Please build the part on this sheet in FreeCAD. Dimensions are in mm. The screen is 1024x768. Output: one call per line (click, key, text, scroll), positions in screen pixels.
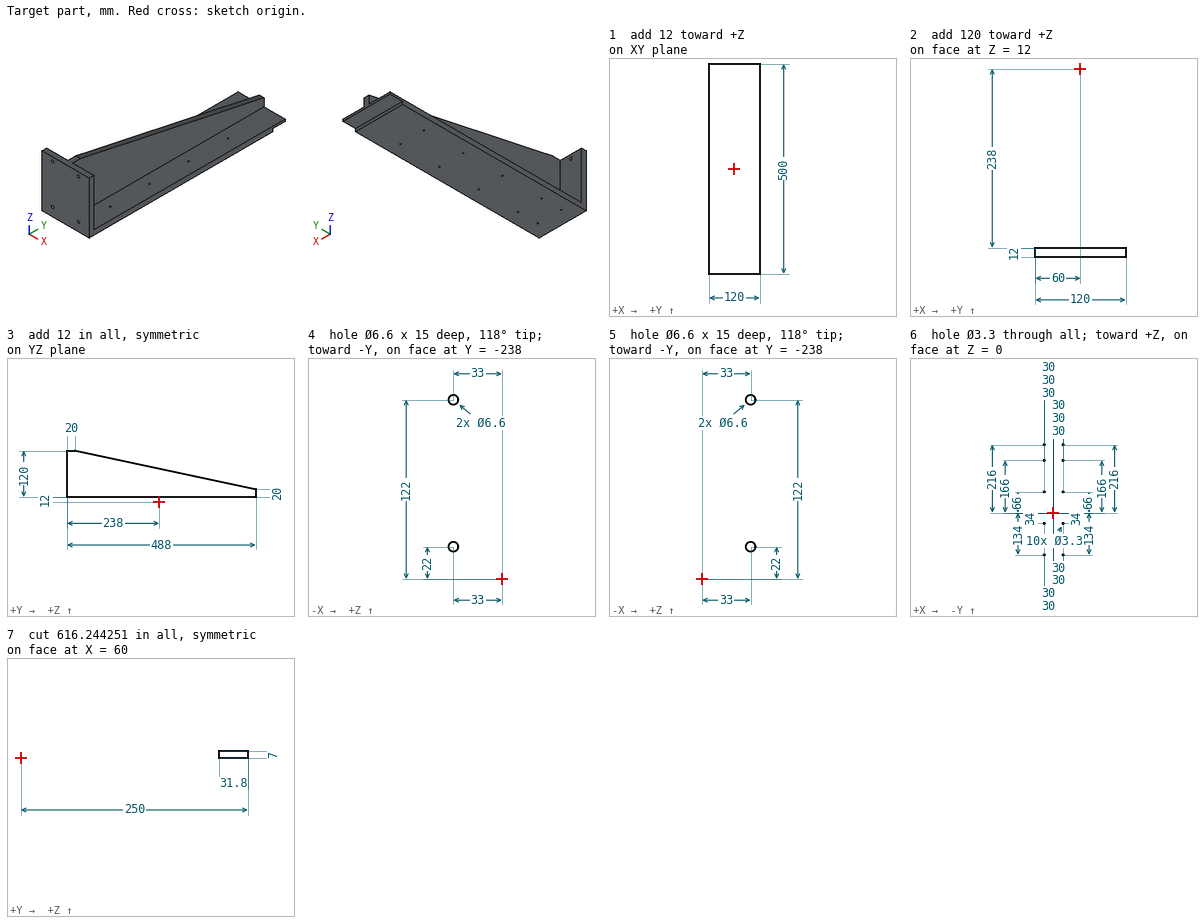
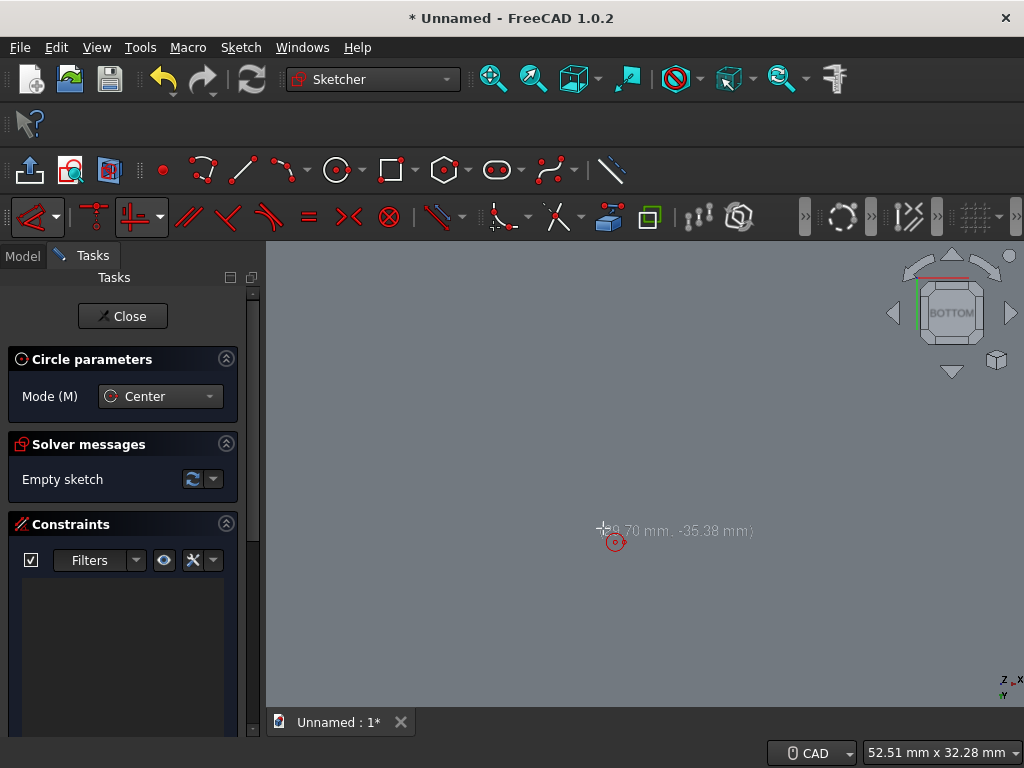
scroll(603, 541, down, 14)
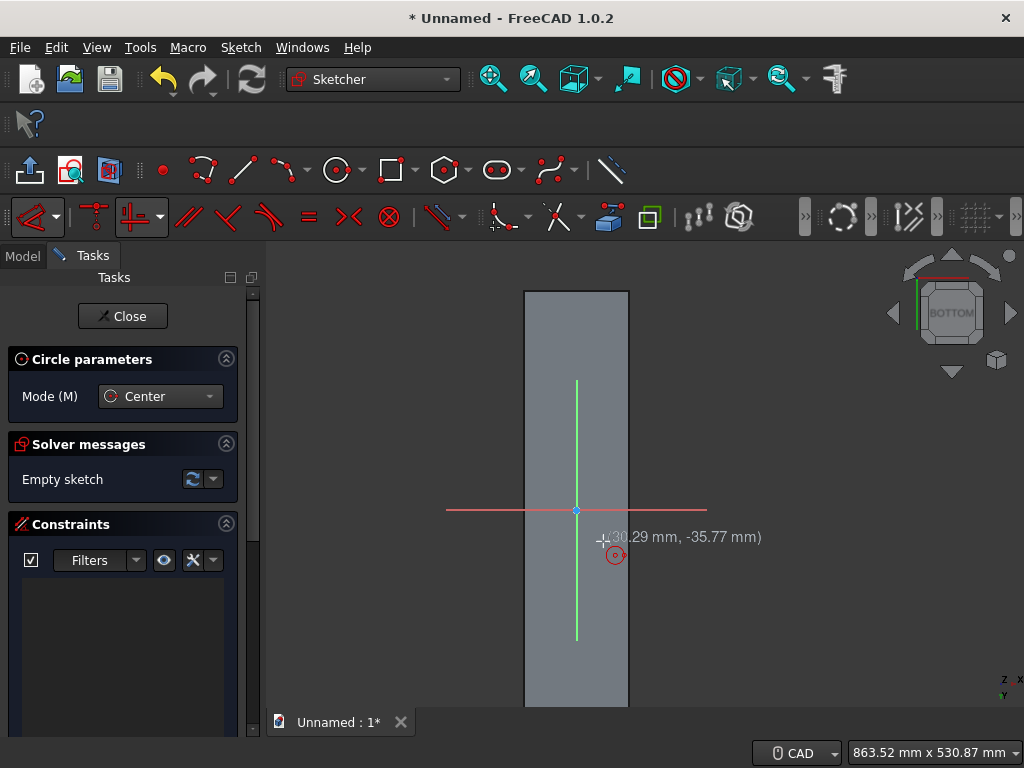
click(603, 540)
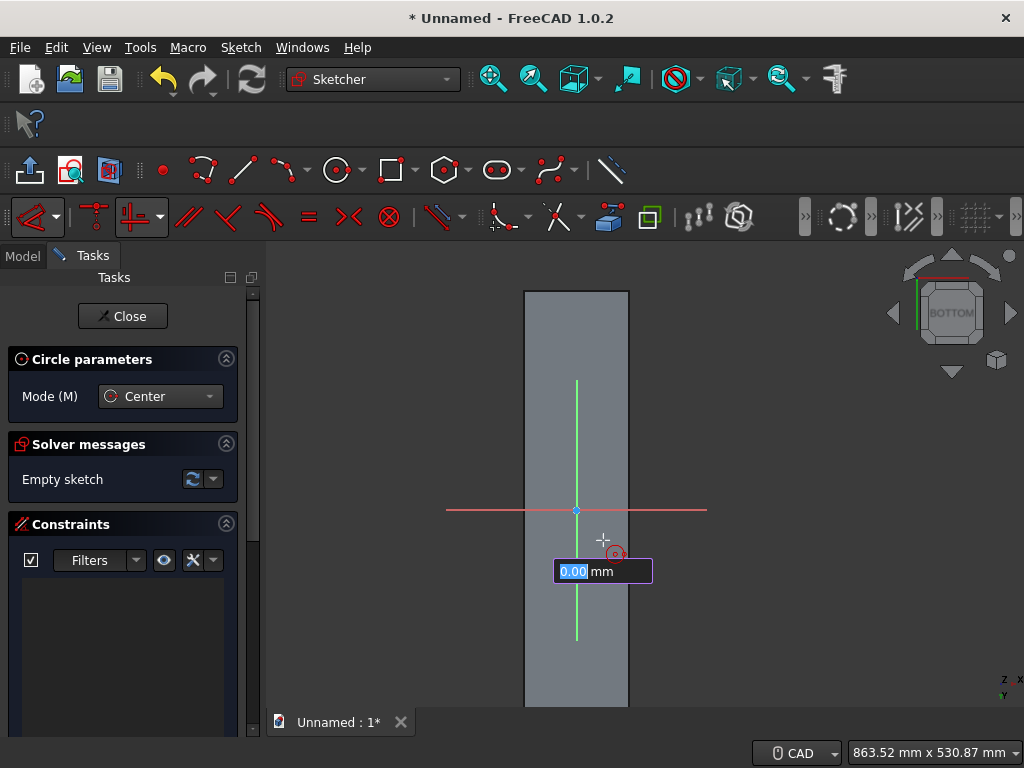
scroll(604, 539, up, 12)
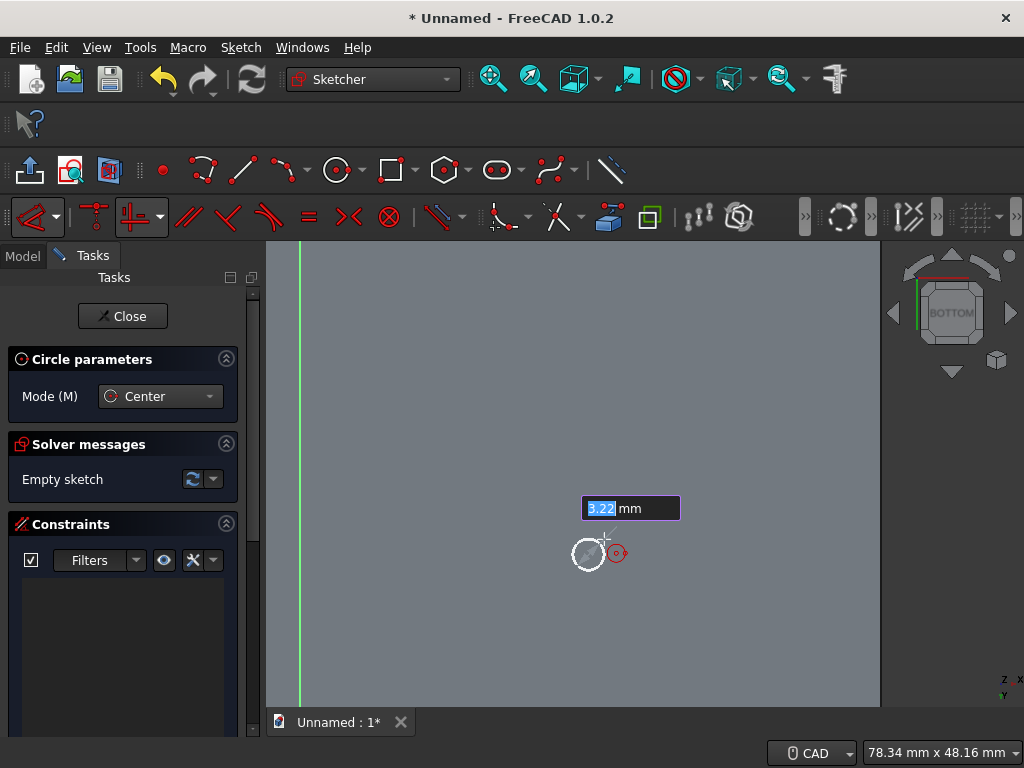
click(602, 534)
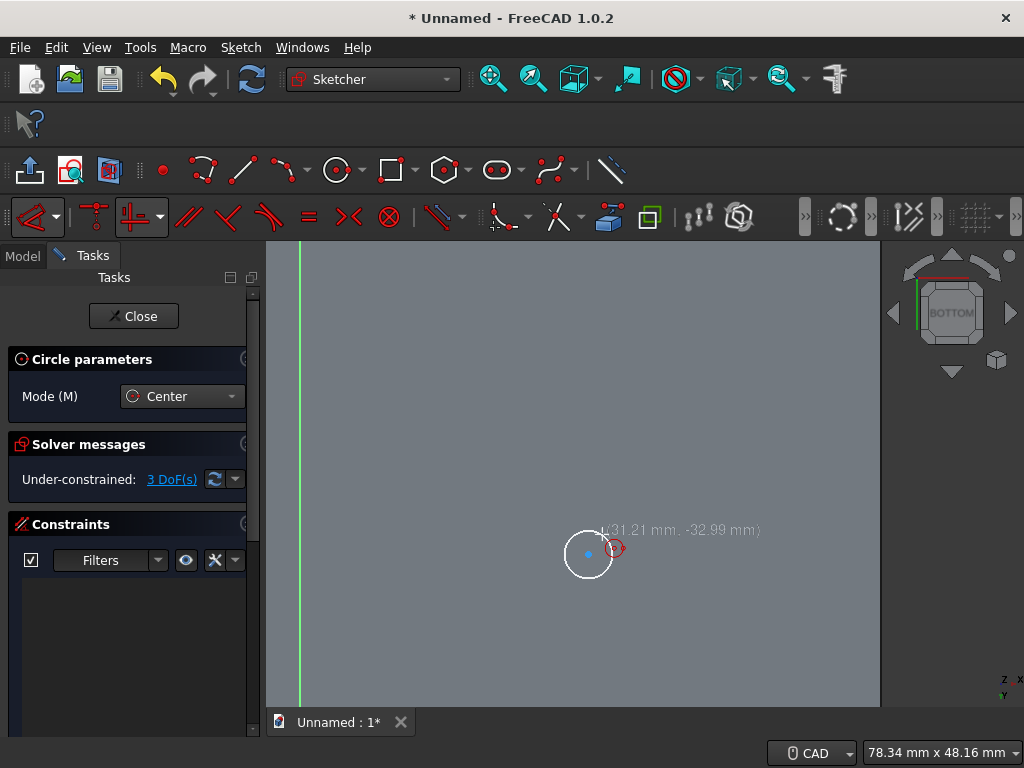
scroll(604, 539, down, 12)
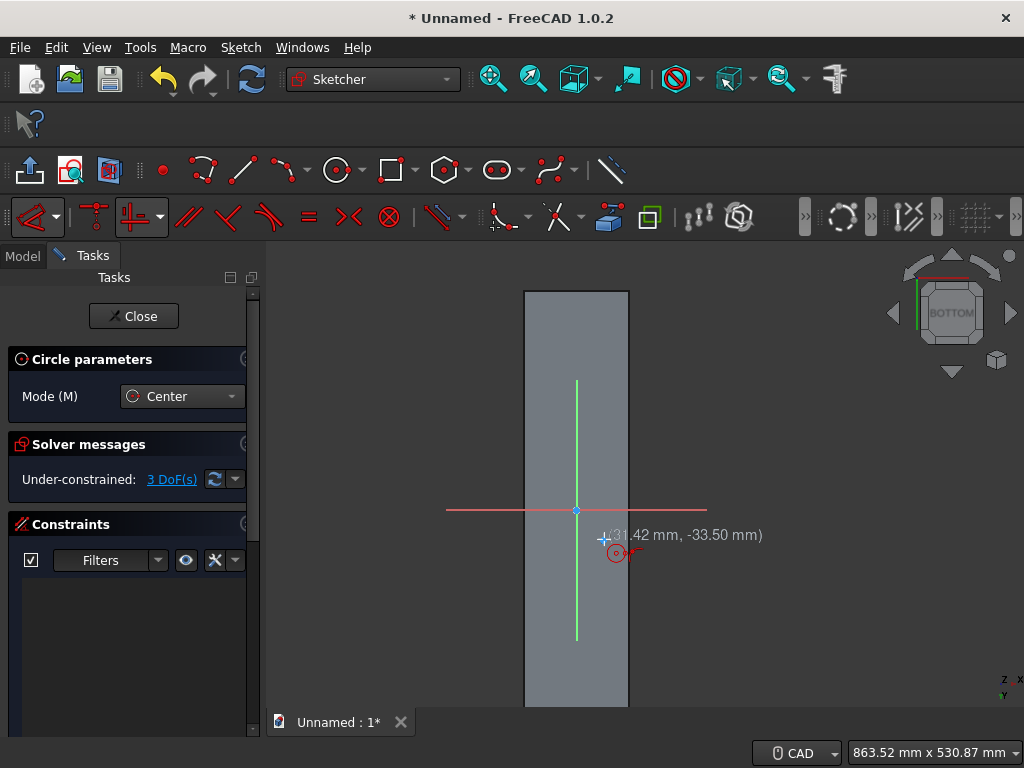
scroll(603, 628, up, 14)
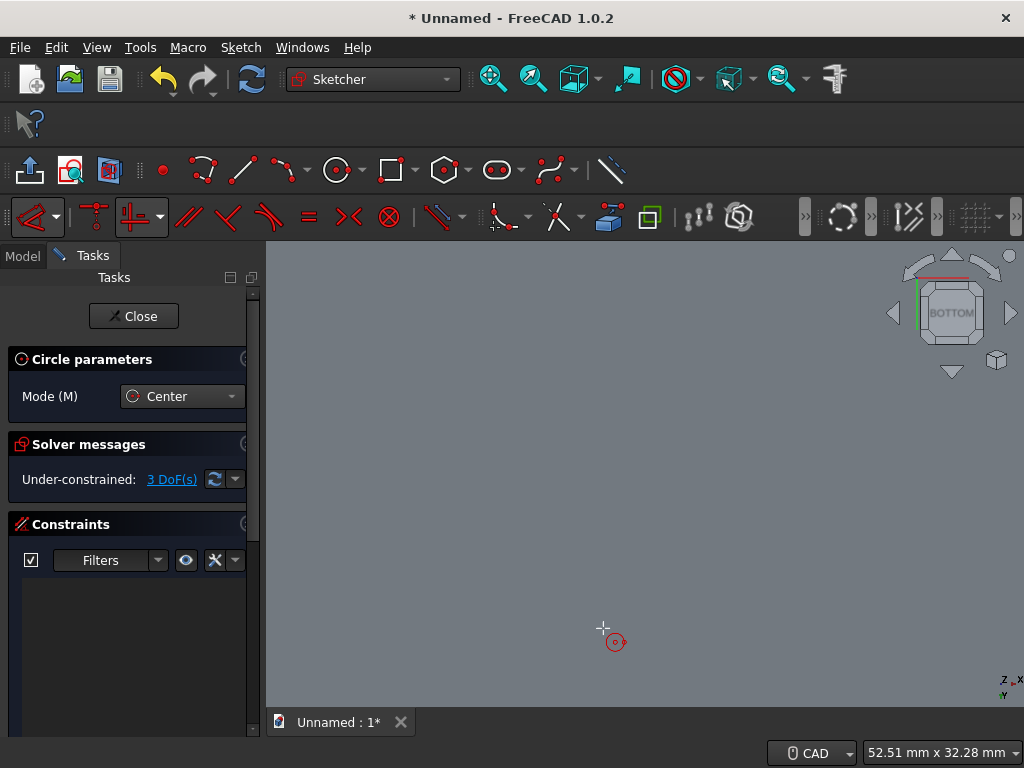
scroll(603, 629, down, 14)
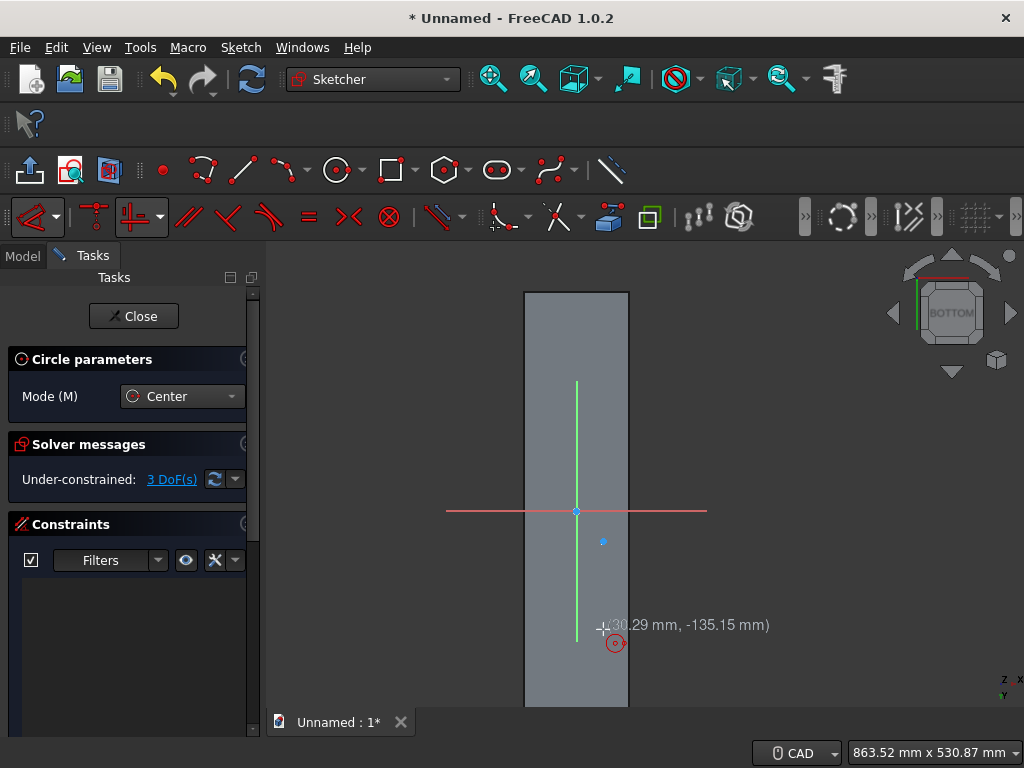
click(603, 629)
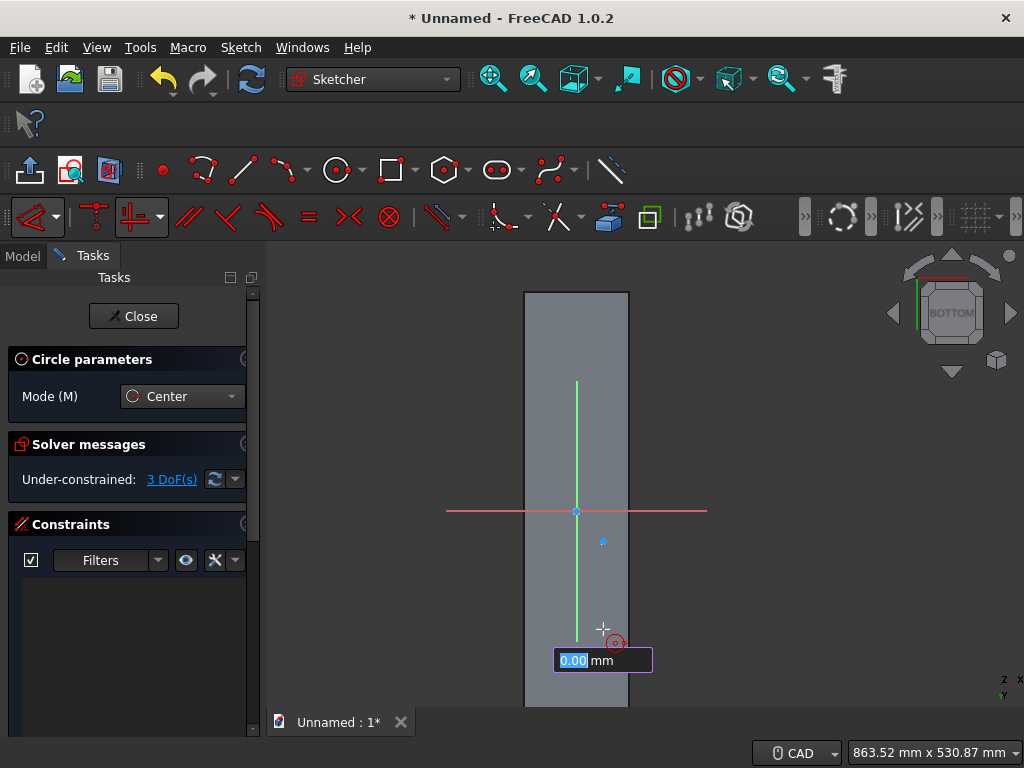
scroll(604, 628, up, 12)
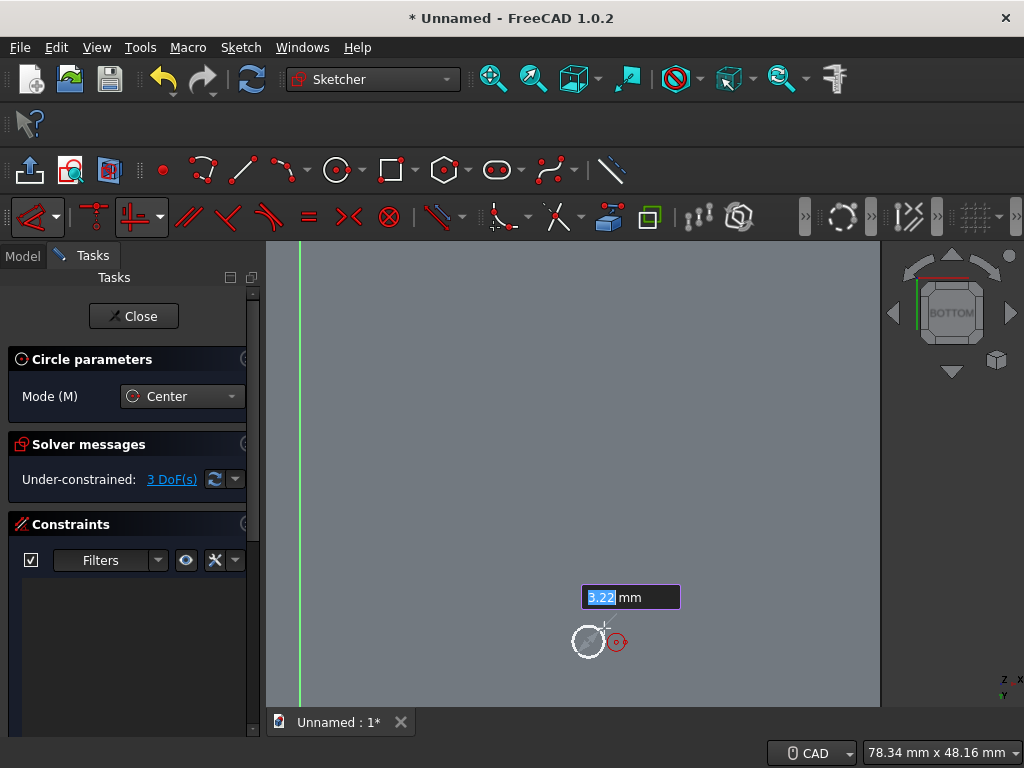
click(602, 618)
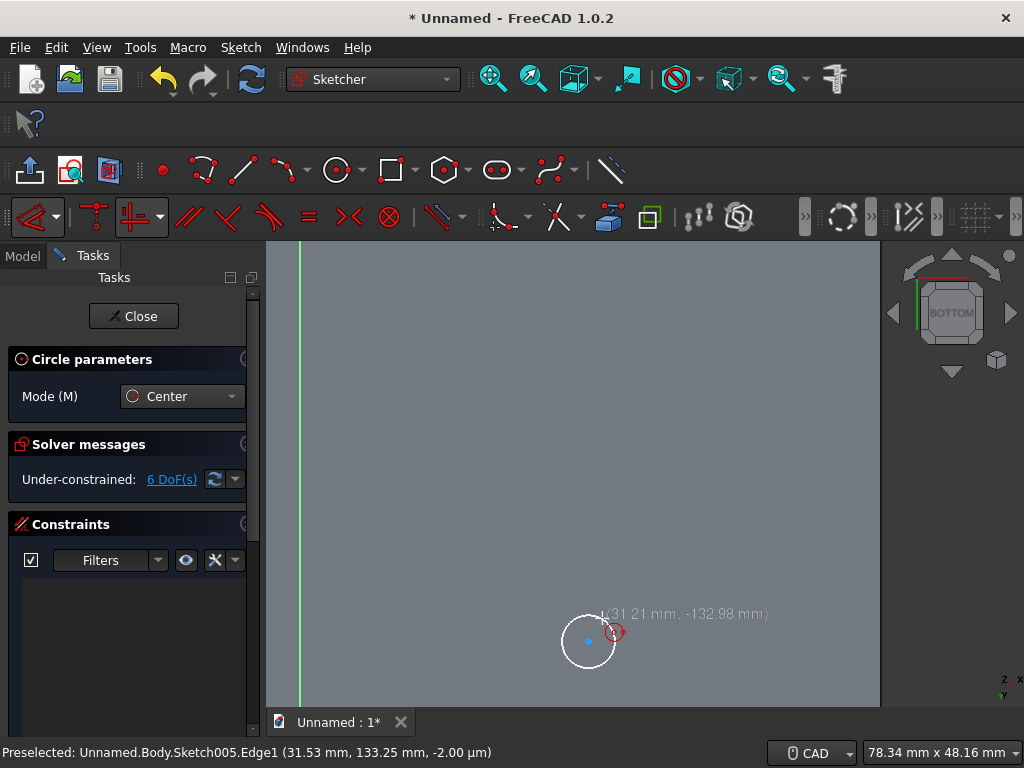
scroll(604, 627, down, 12)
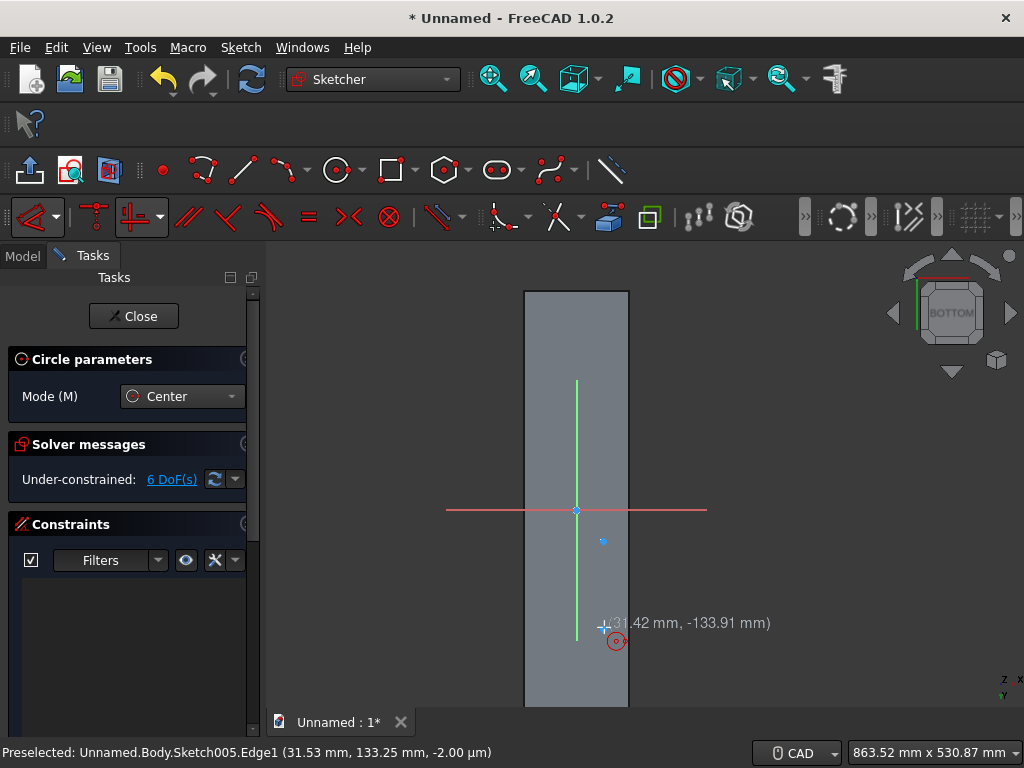
scroll(603, 452, up, 14)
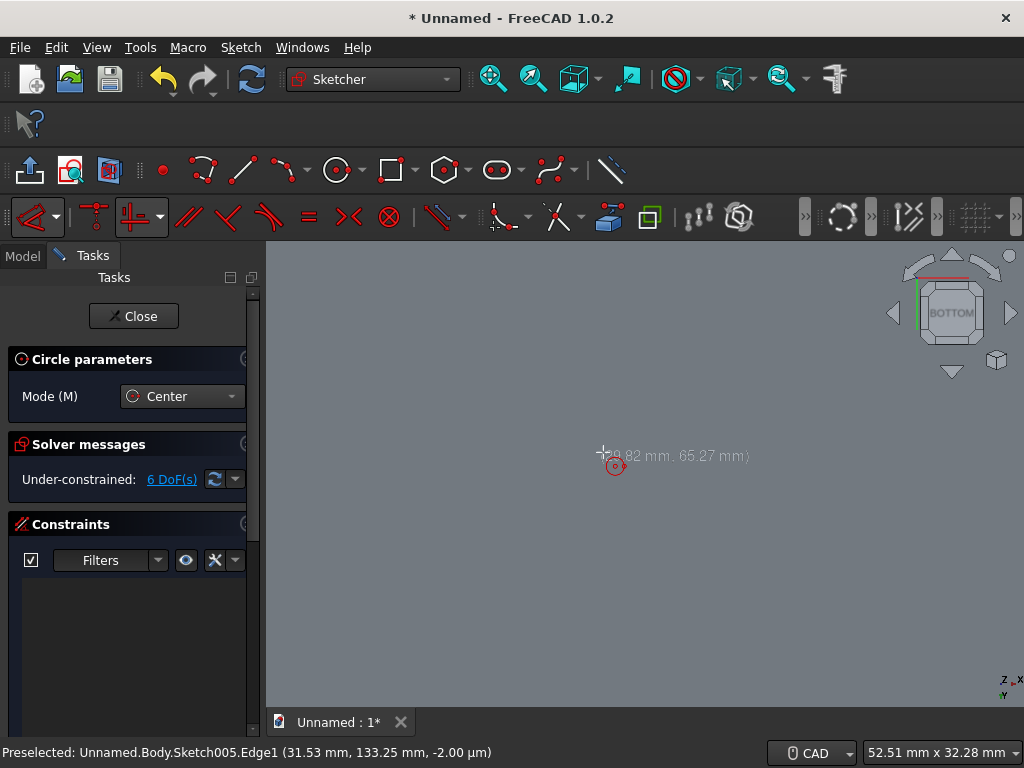
scroll(603, 452, down, 14)